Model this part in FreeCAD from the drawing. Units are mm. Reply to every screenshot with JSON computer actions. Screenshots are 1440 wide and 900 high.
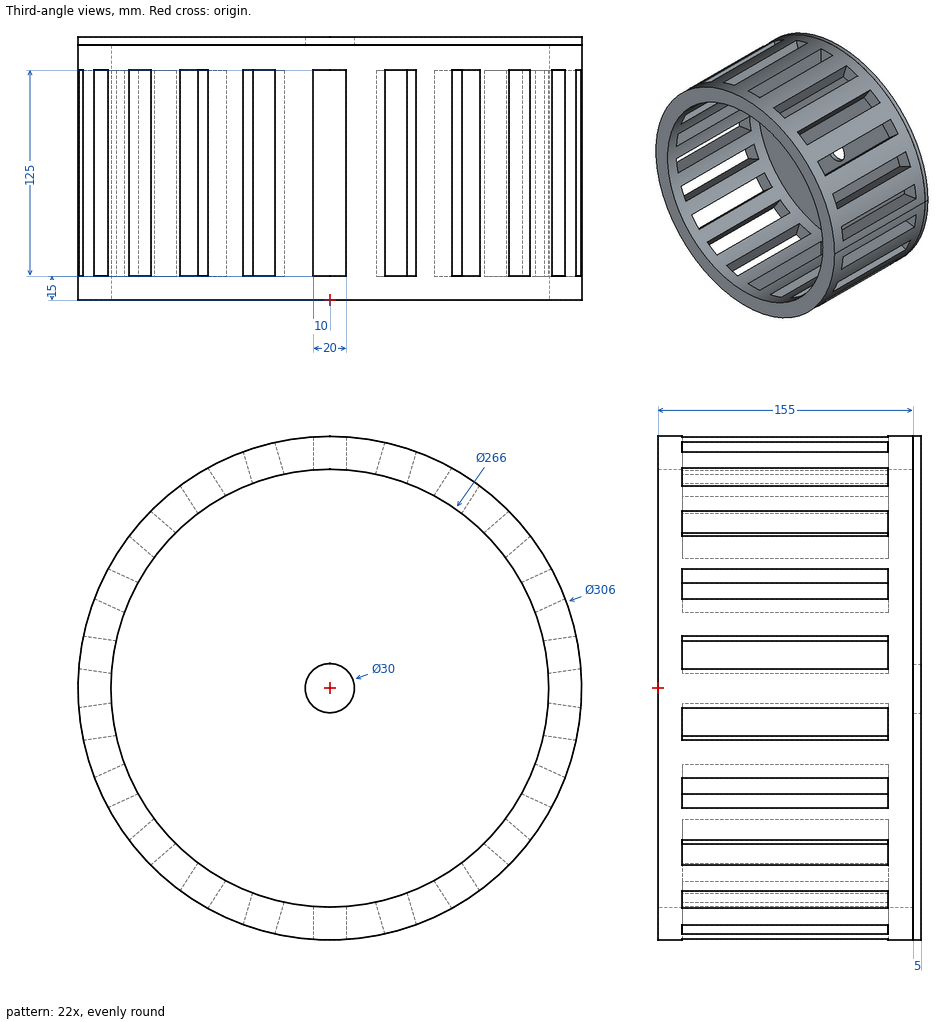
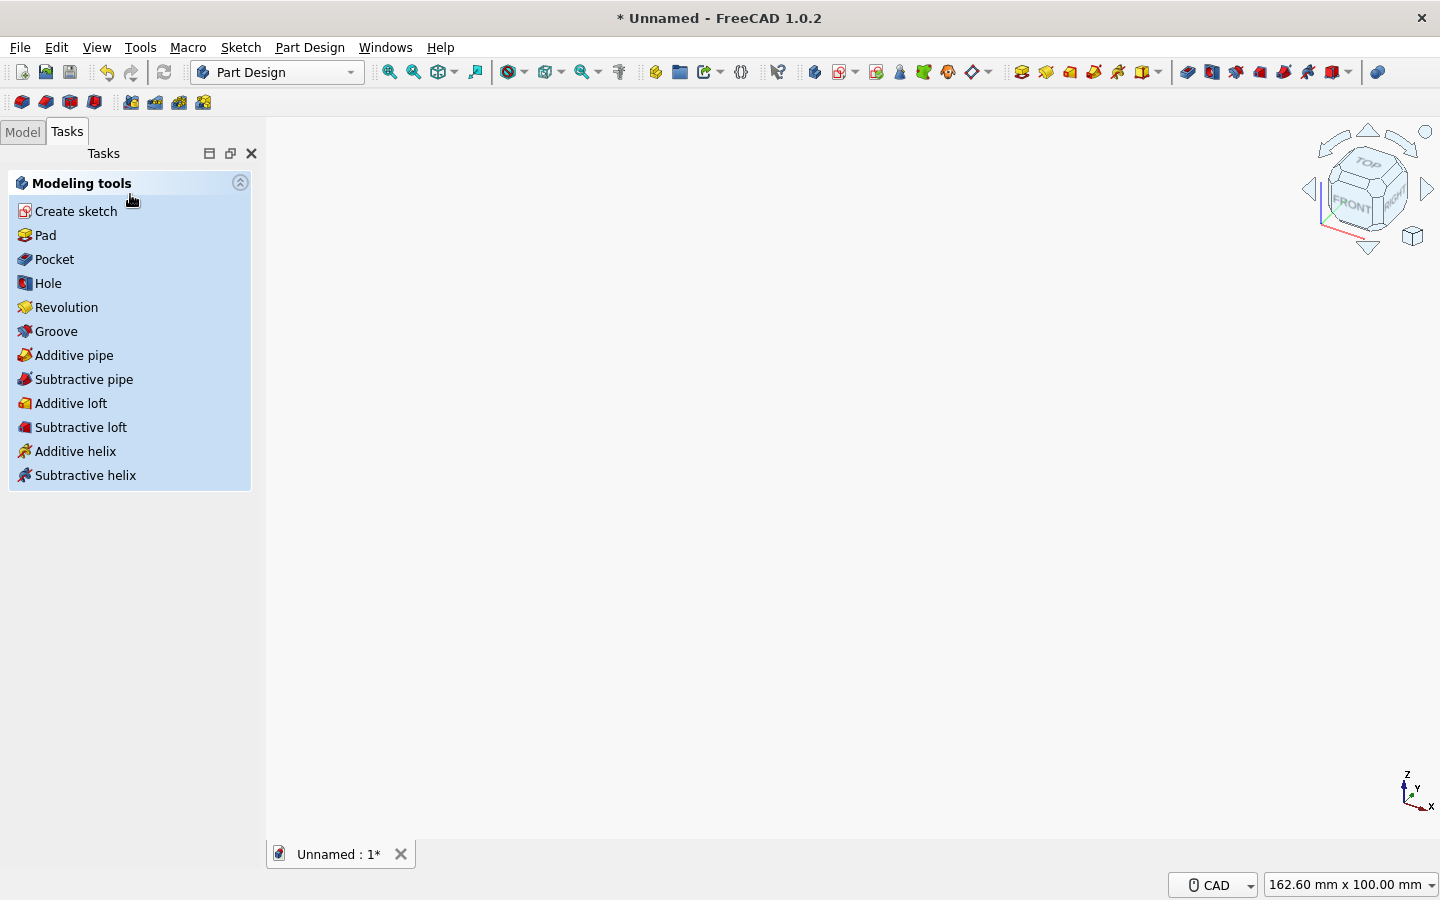
{"action": "left_click", "coordinate": [1022, 72]}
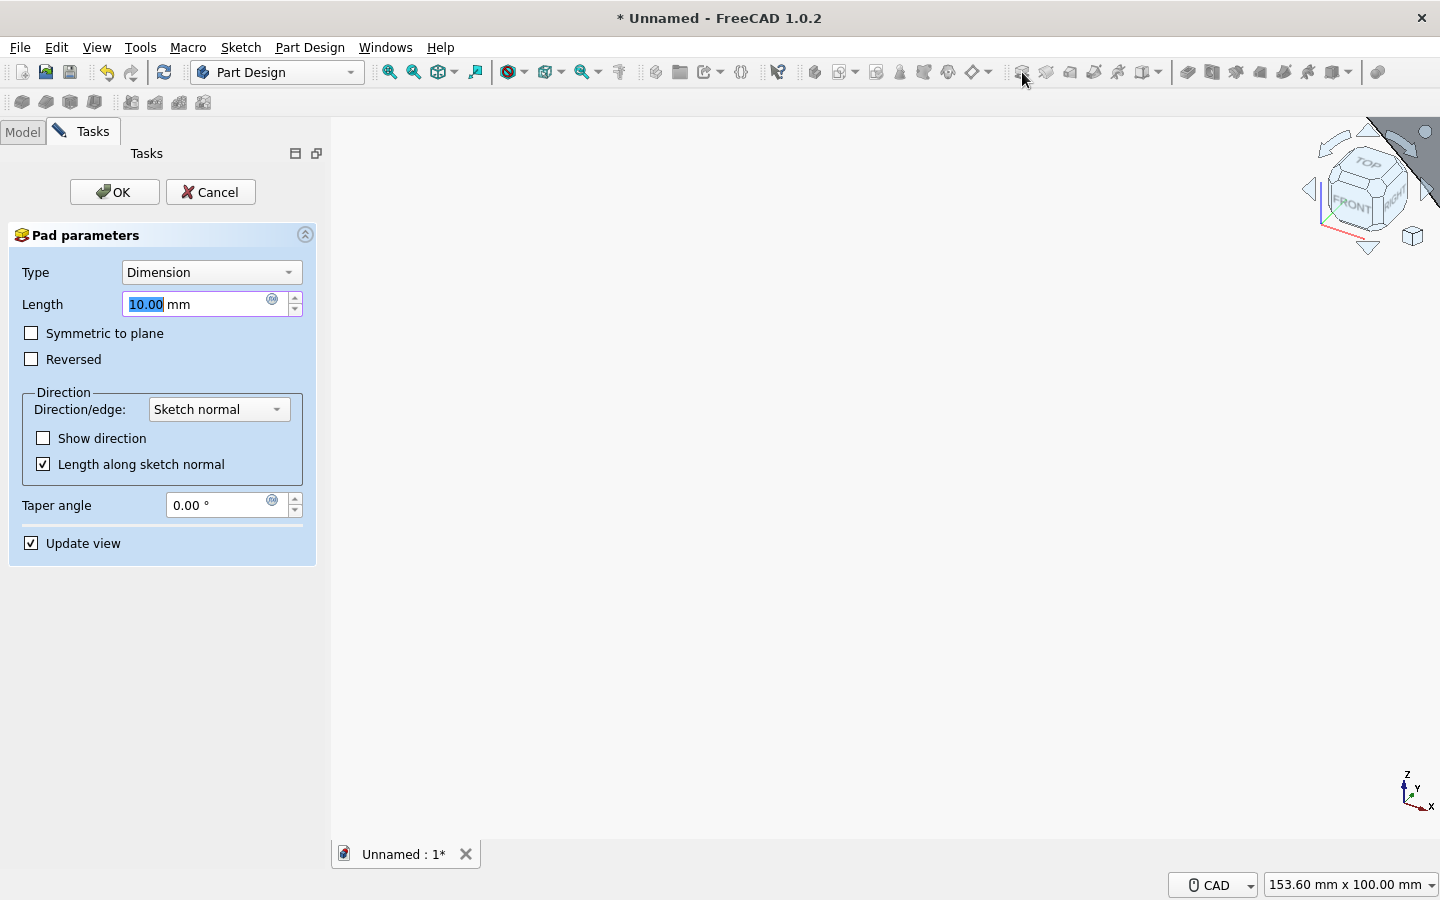
{"action": "type", "text": "155"}
{"action": "key", "text": "Tab"}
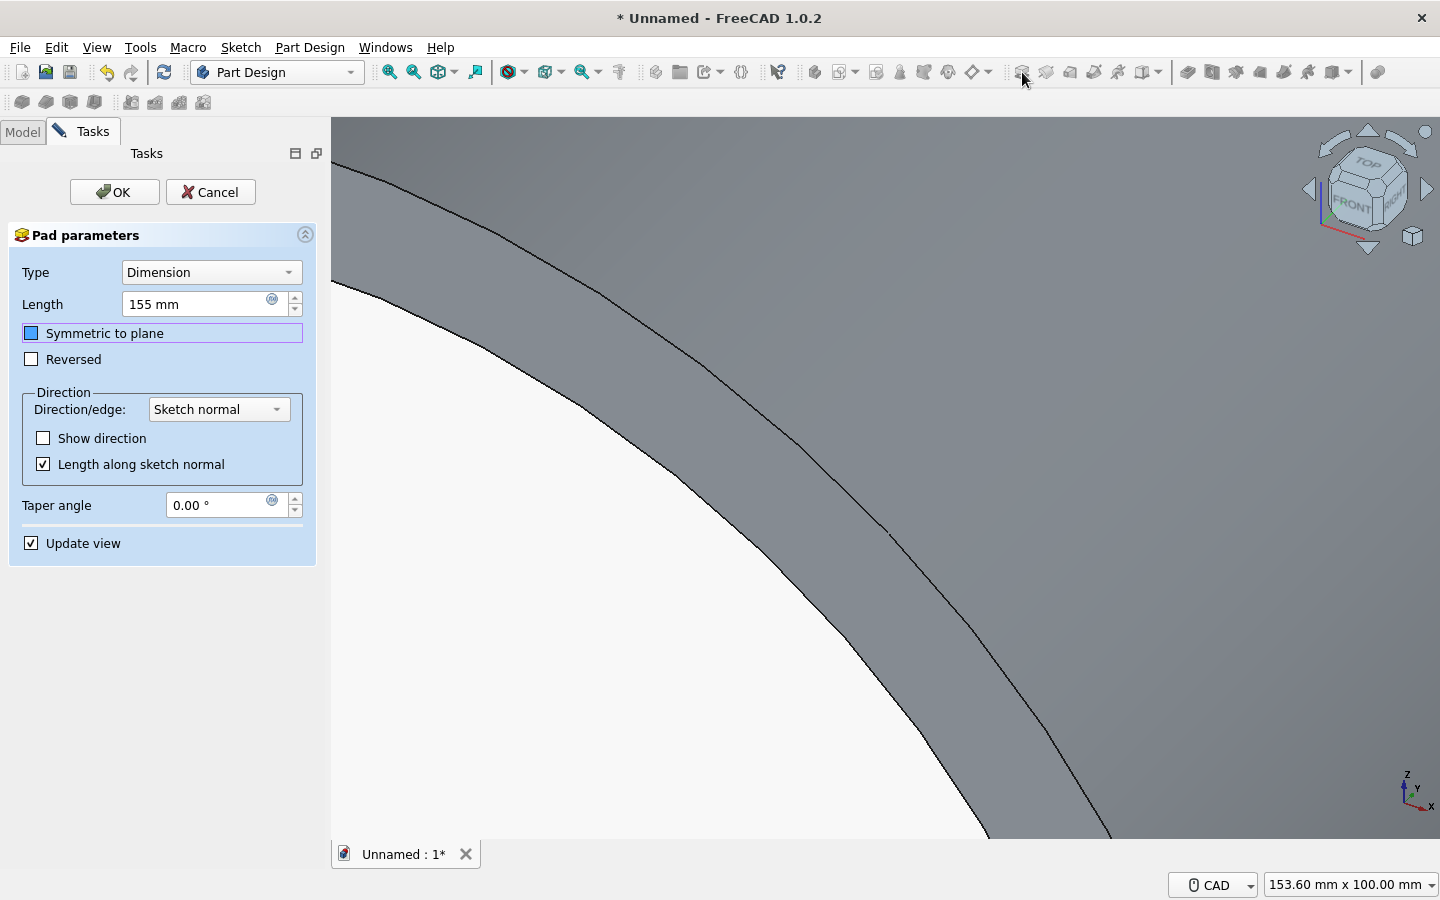
{"action": "left_click", "coordinate": [30, 359]}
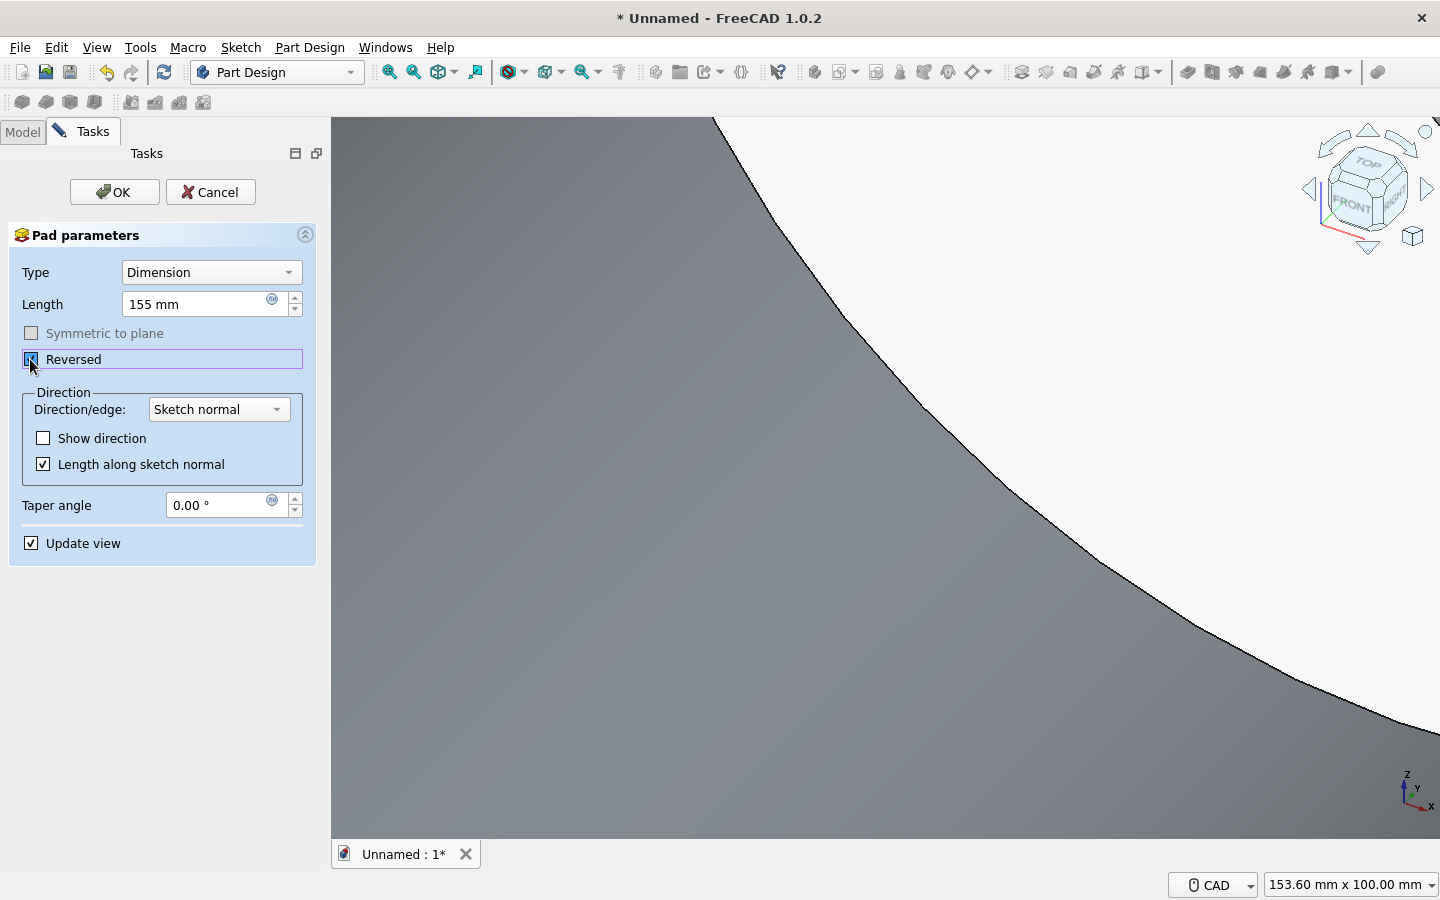
{"action": "left_click", "coordinate": [115, 192]}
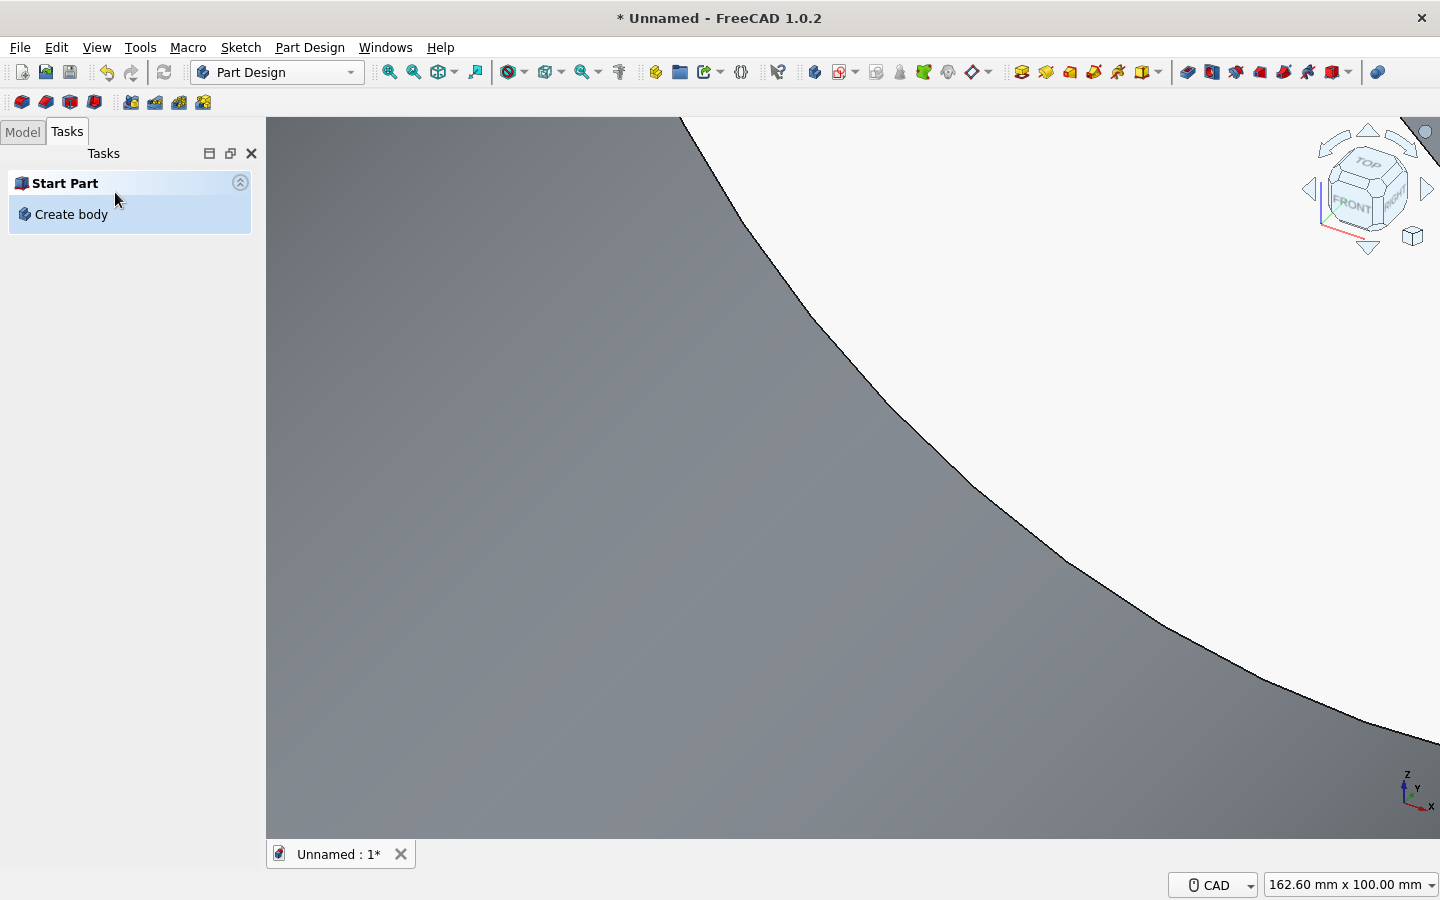
{"action": "left_click", "coordinate": [390, 72]}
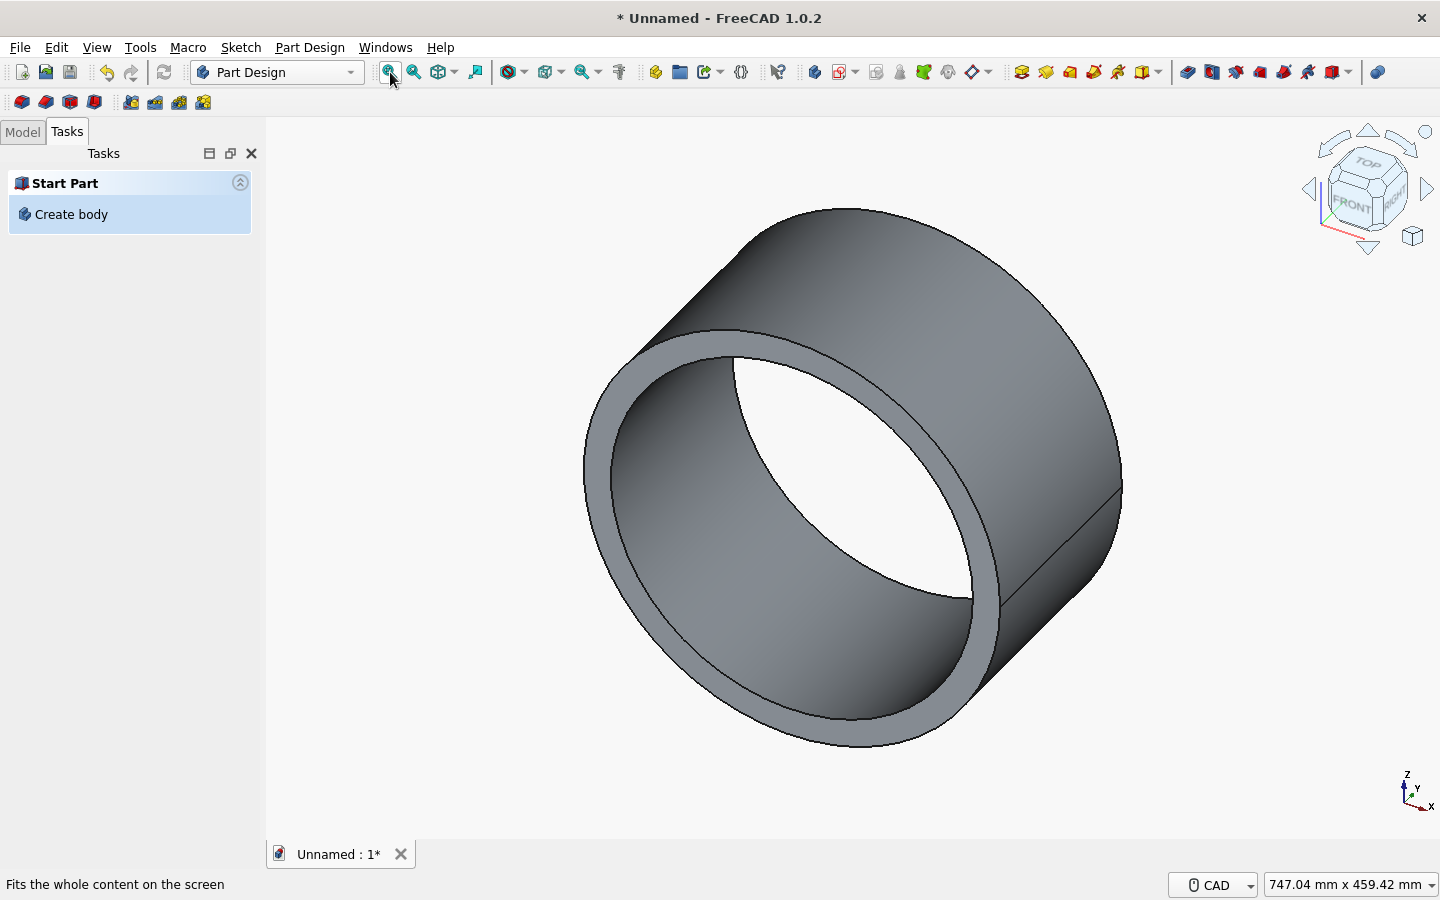
{"action": "left_click", "coordinate": [840, 72]}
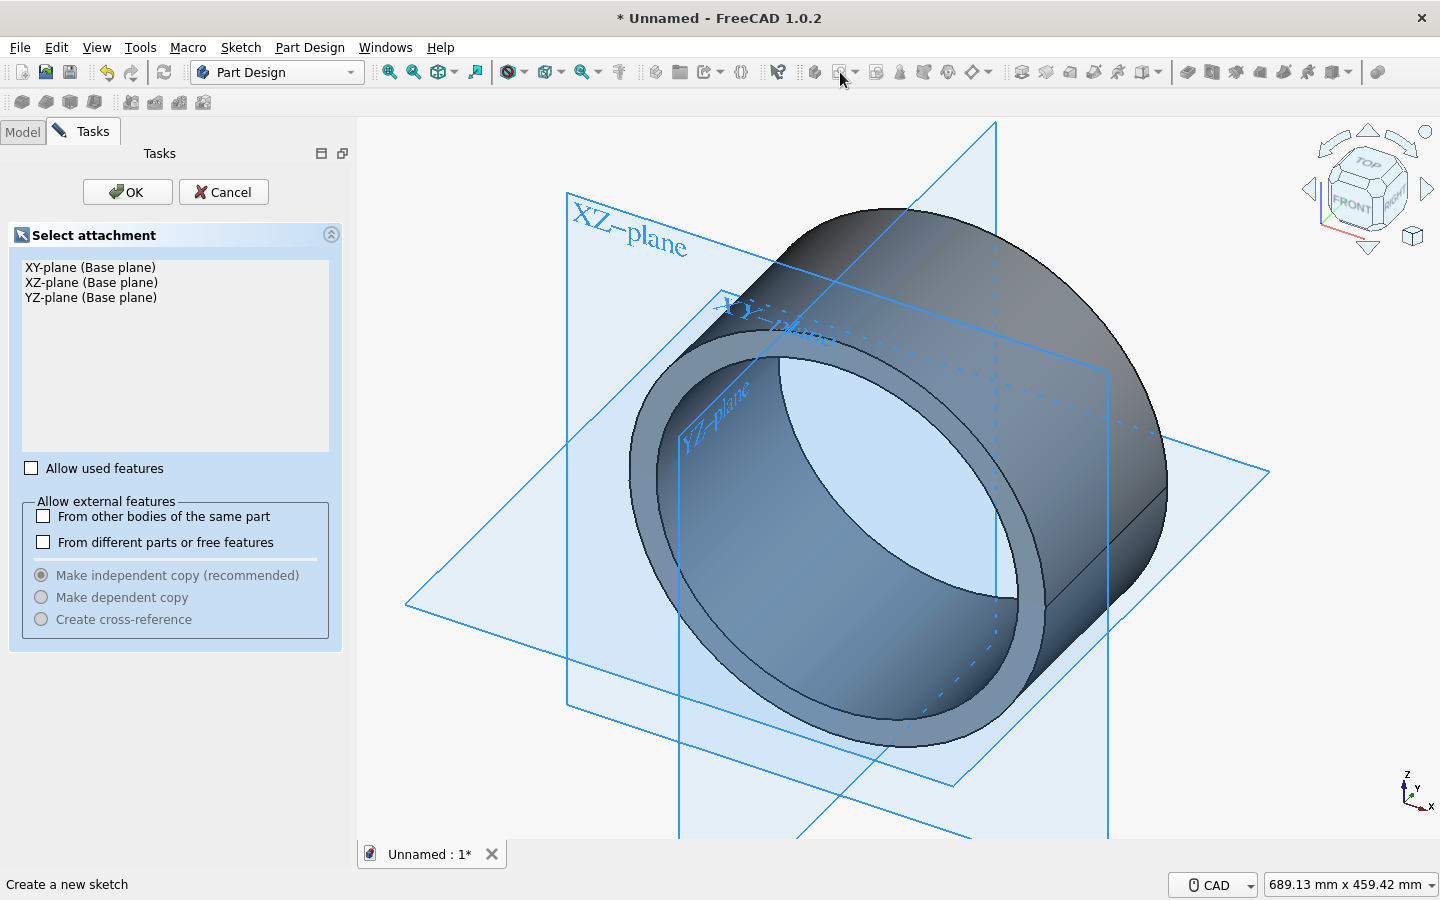
{"action": "left_click", "coordinate": [82, 268]}